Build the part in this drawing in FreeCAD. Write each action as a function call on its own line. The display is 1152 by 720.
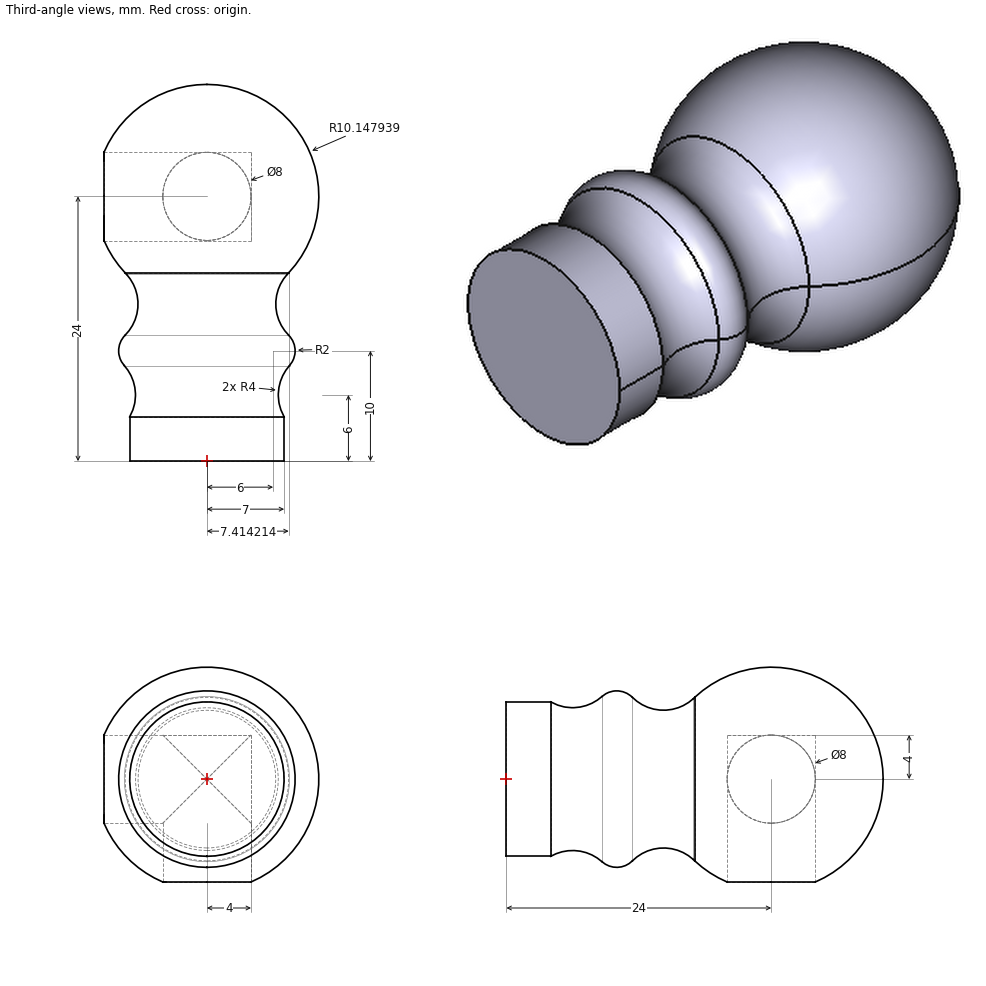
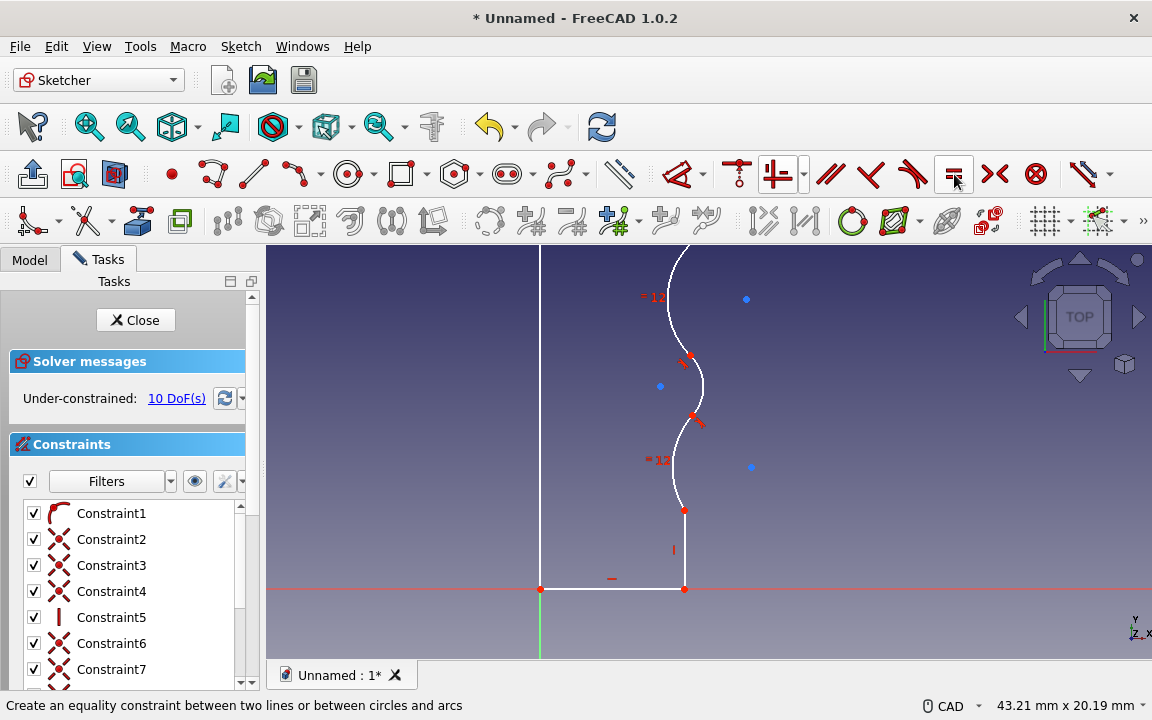
scroll(643, 576, down, 5)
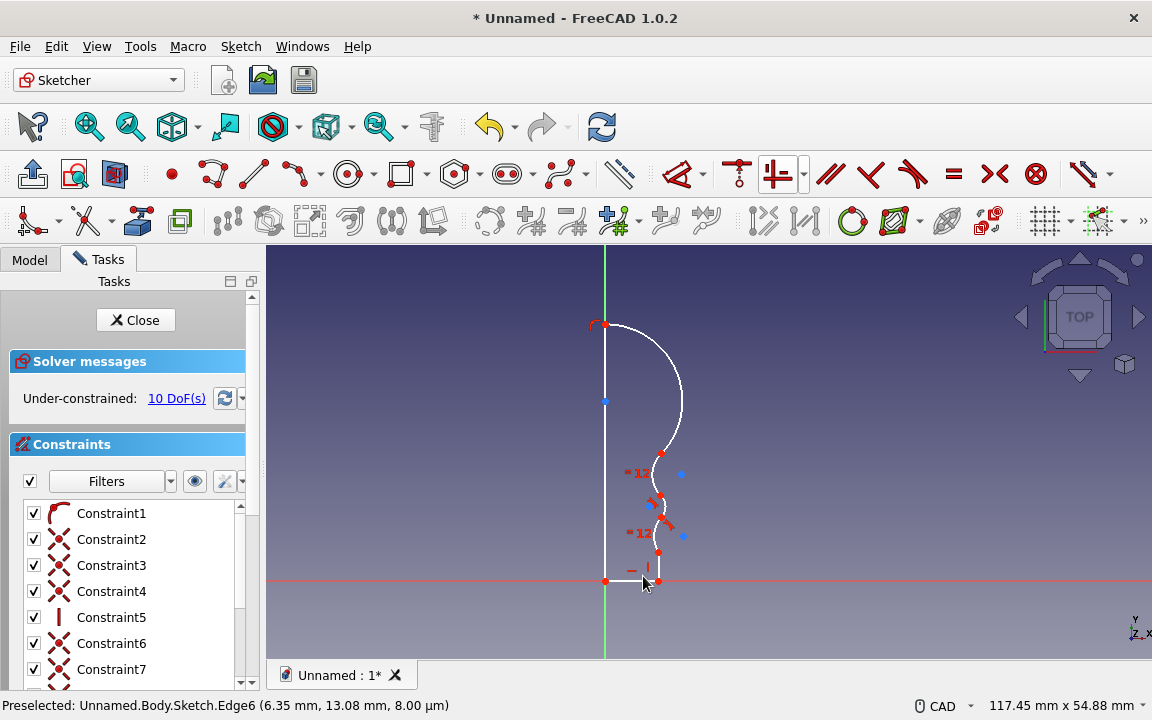
click(606, 401)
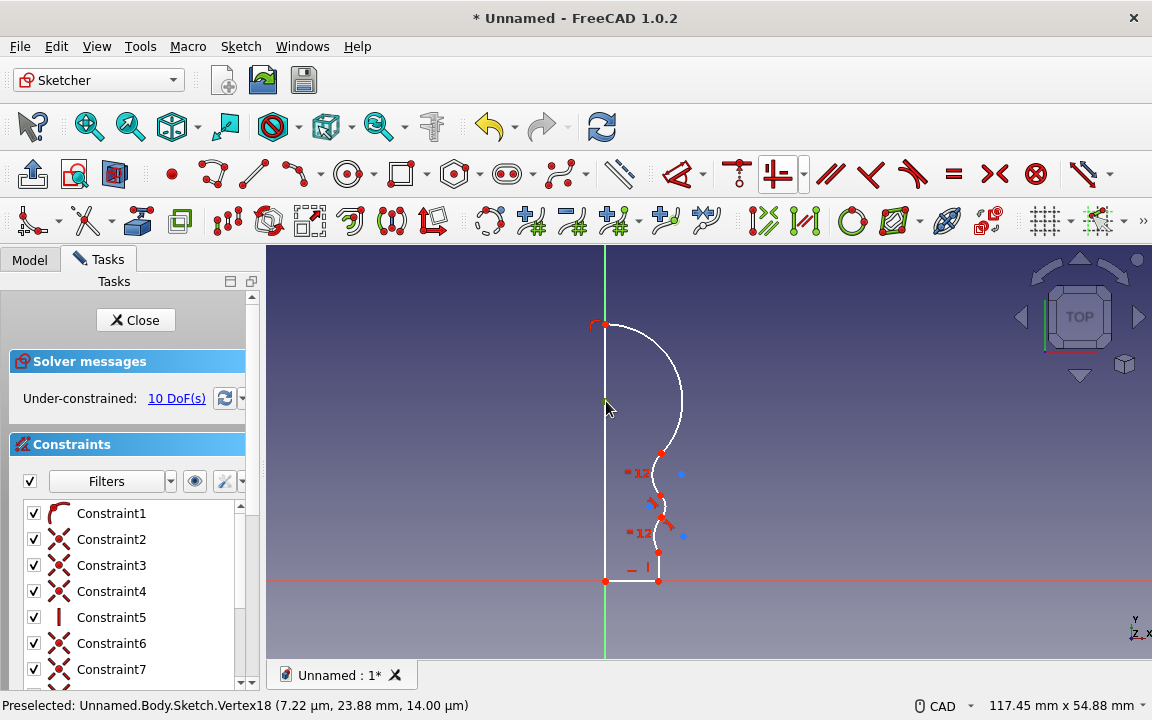
click(605, 299)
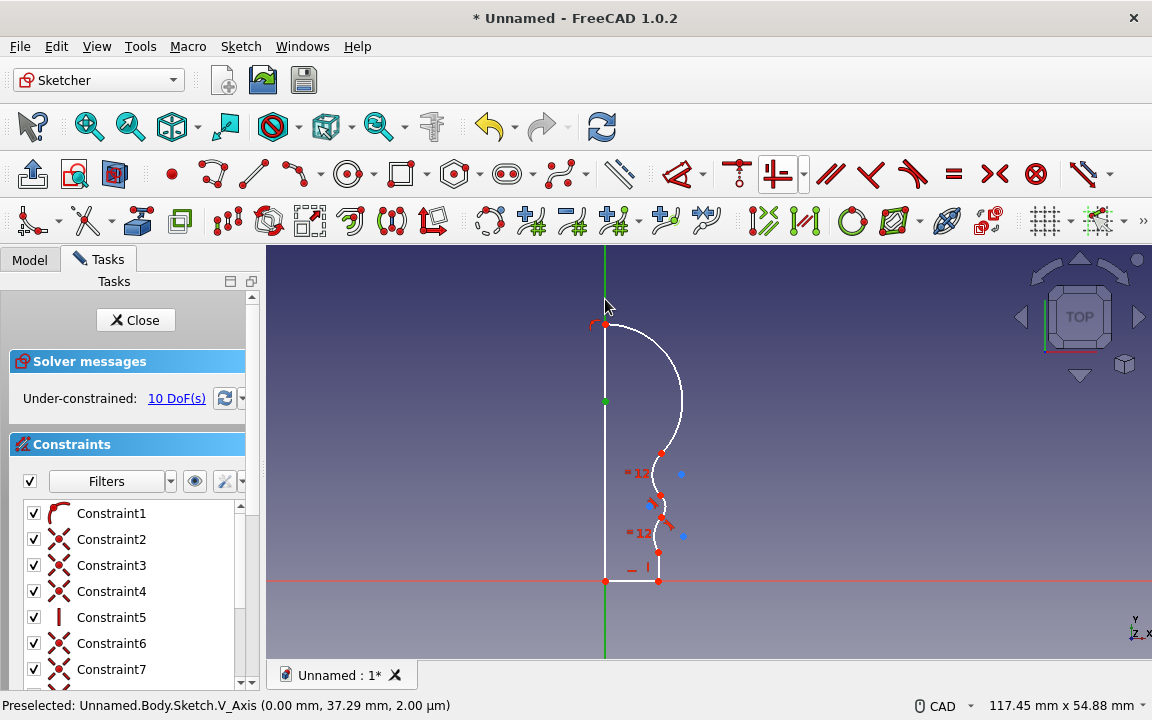
click(737, 174)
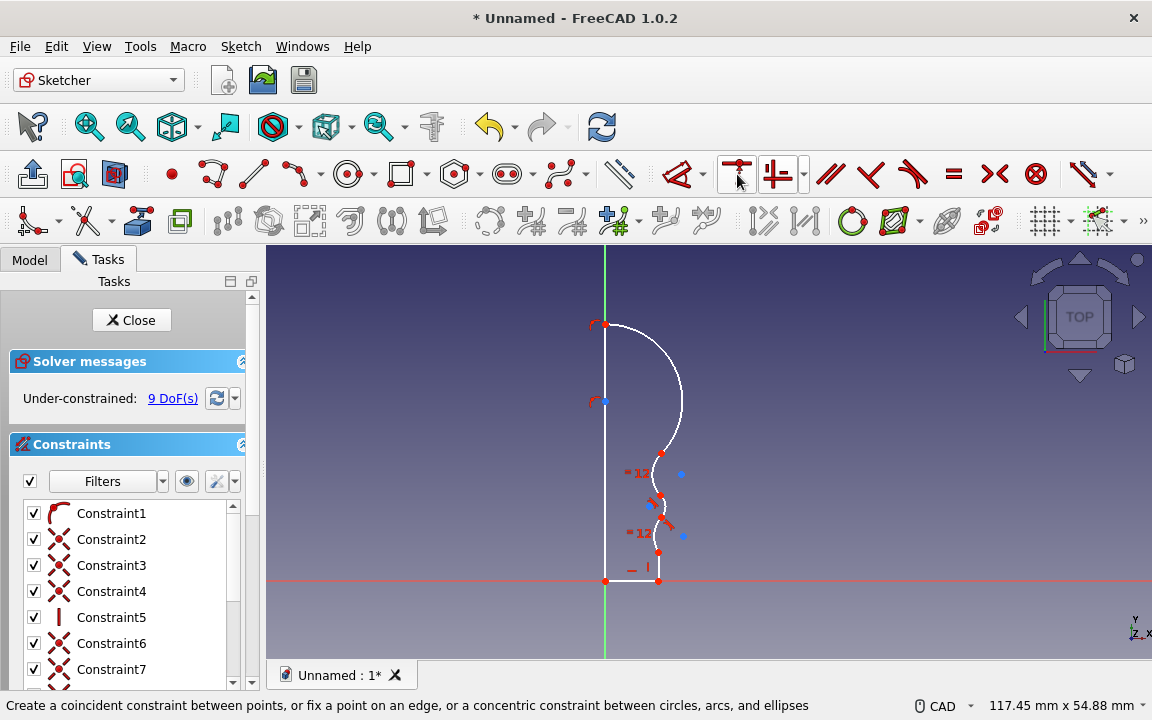
scroll(656, 527, up, 2)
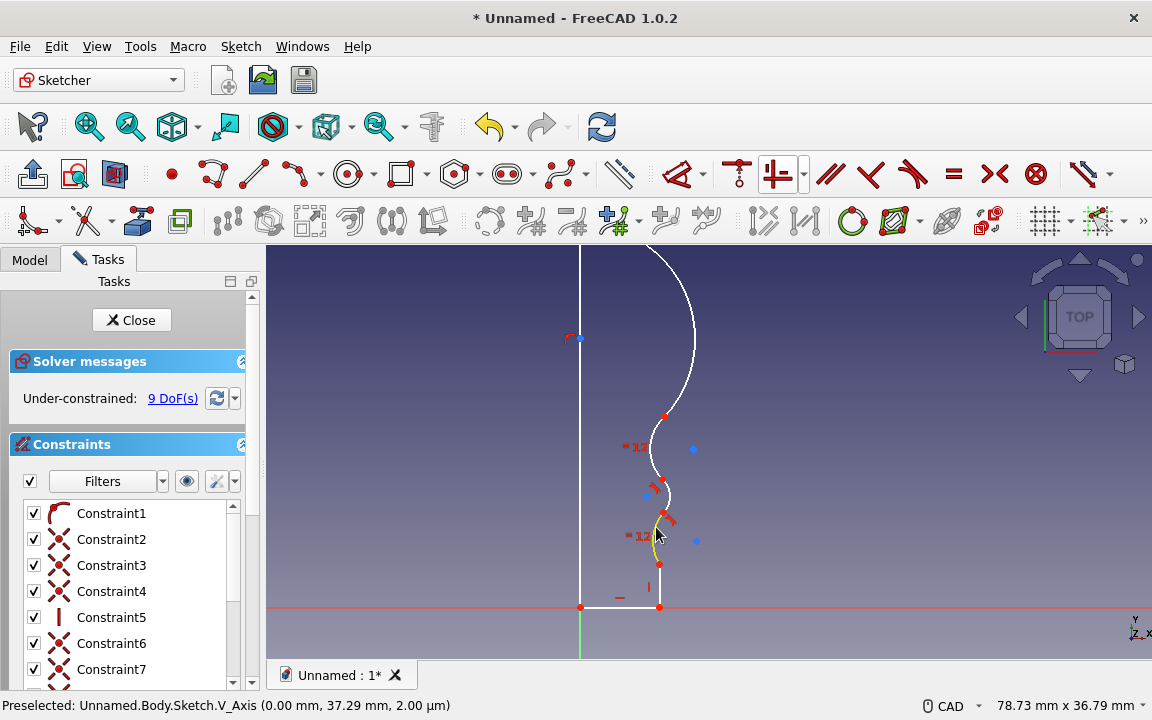
click(656, 527)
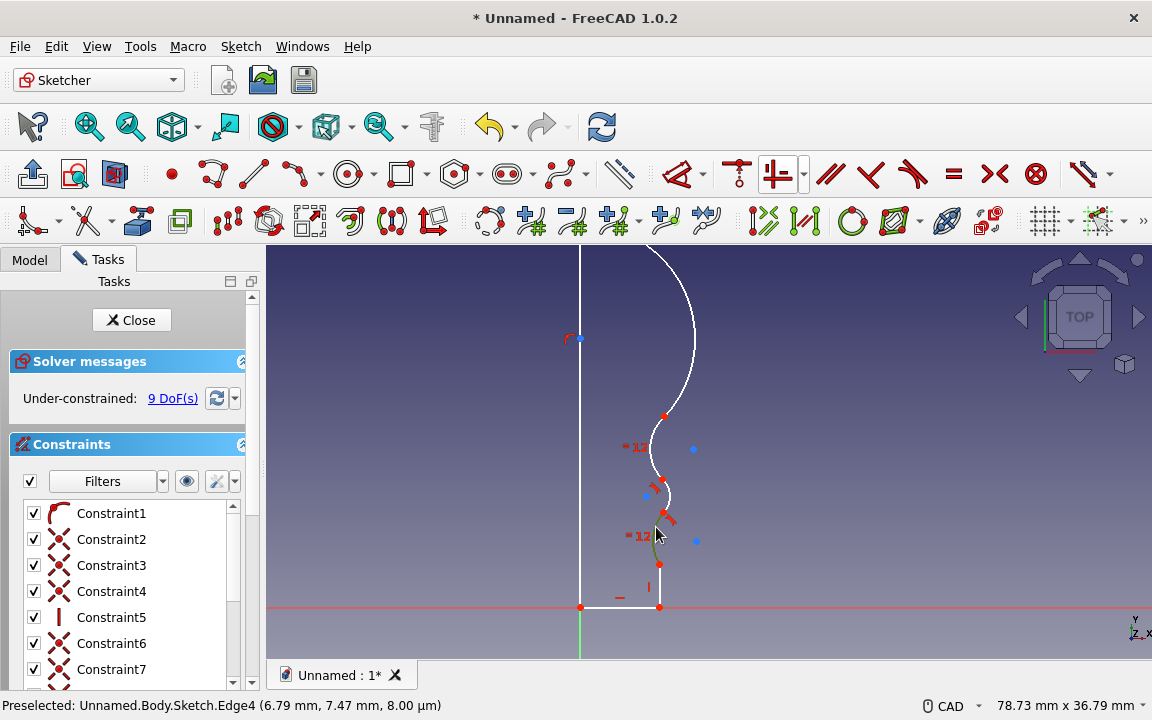
key(k)
key(r)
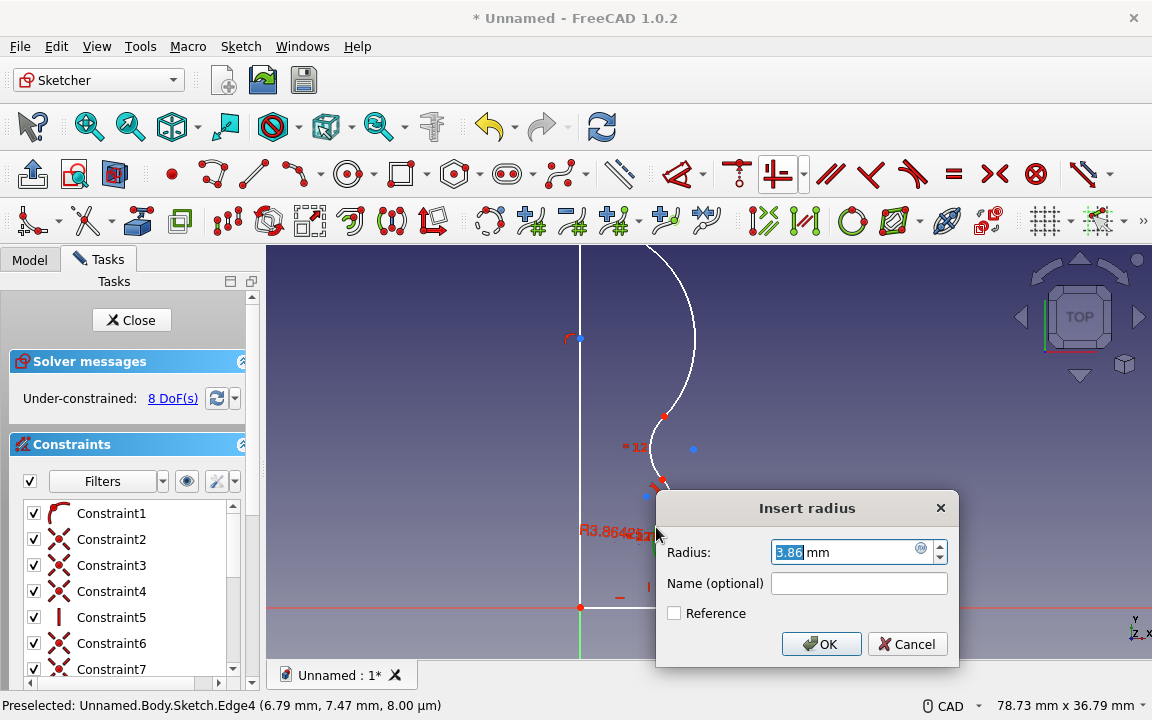
text(4)
key(Return)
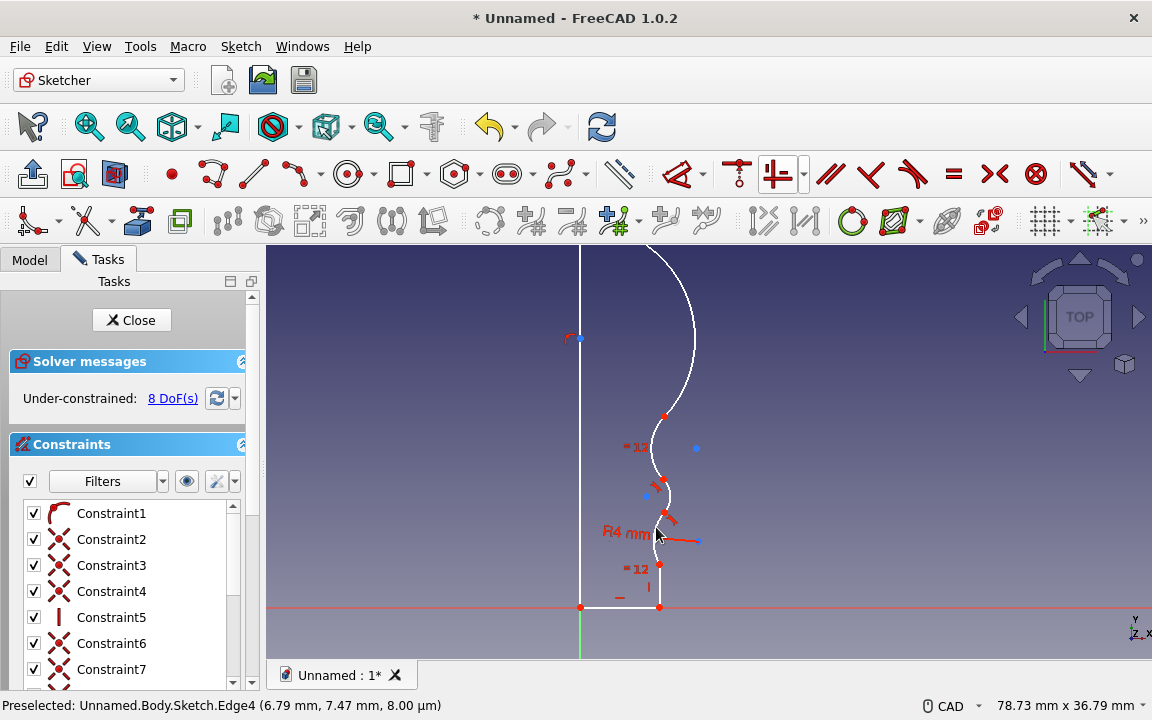
scroll(670, 503, up, 3)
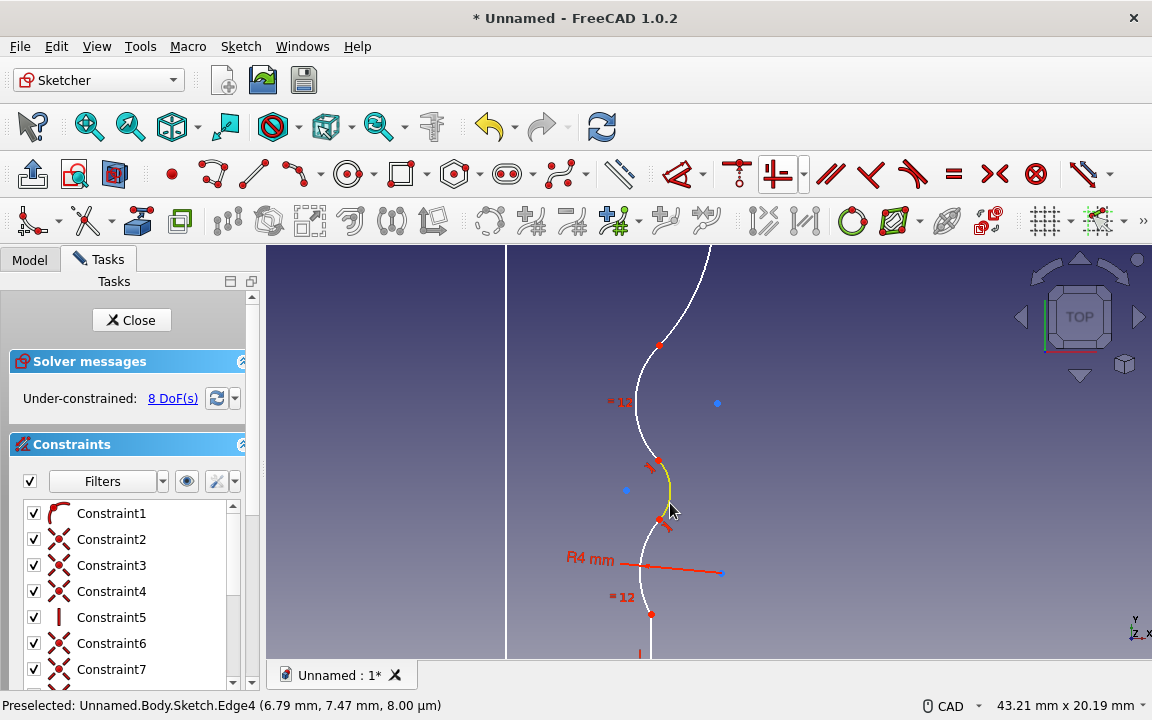
click(669, 502)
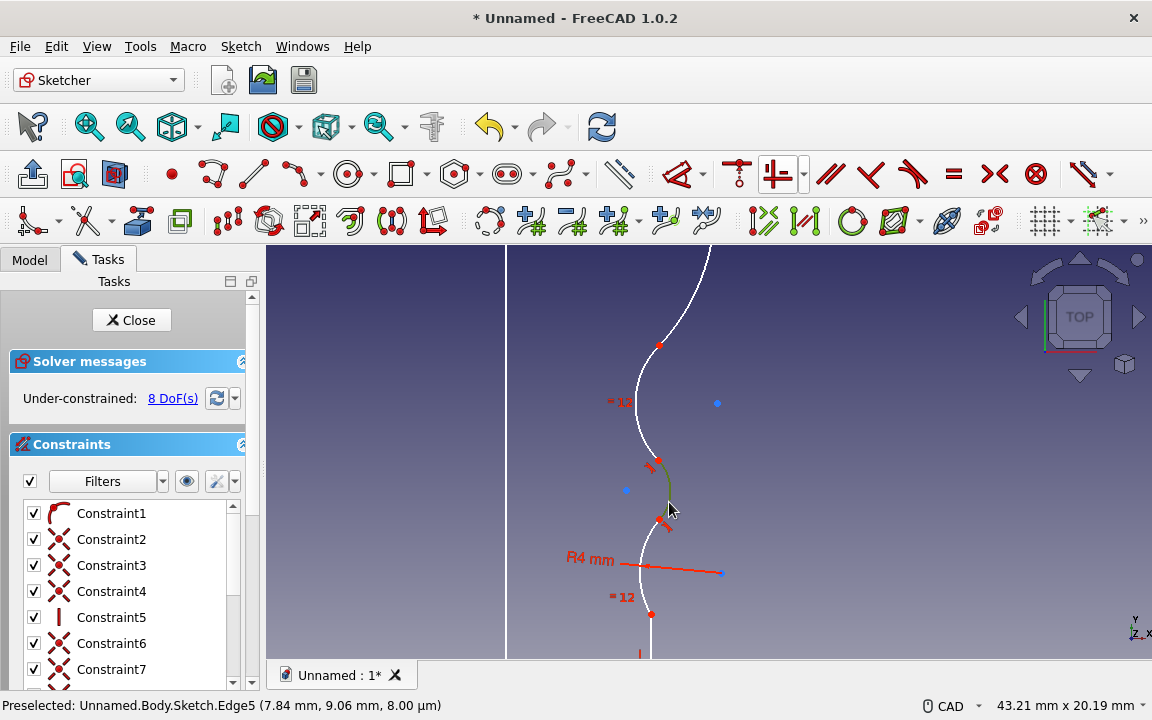
key(k)
key(r)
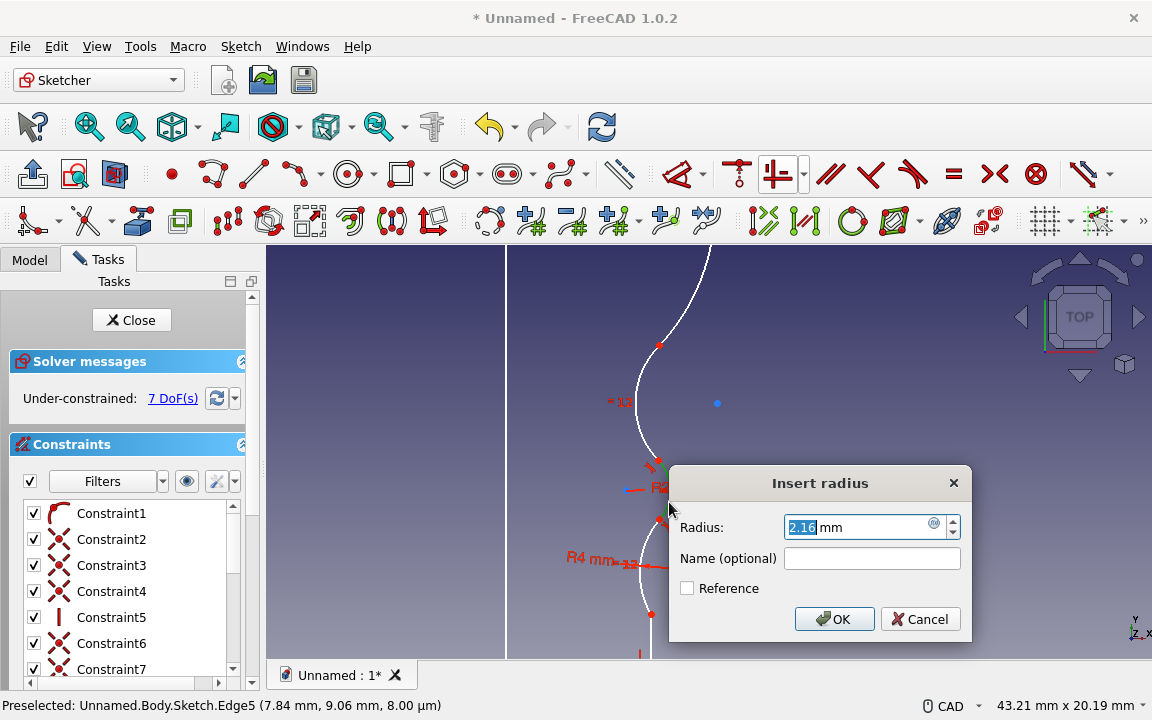
text(2)
key(Return)